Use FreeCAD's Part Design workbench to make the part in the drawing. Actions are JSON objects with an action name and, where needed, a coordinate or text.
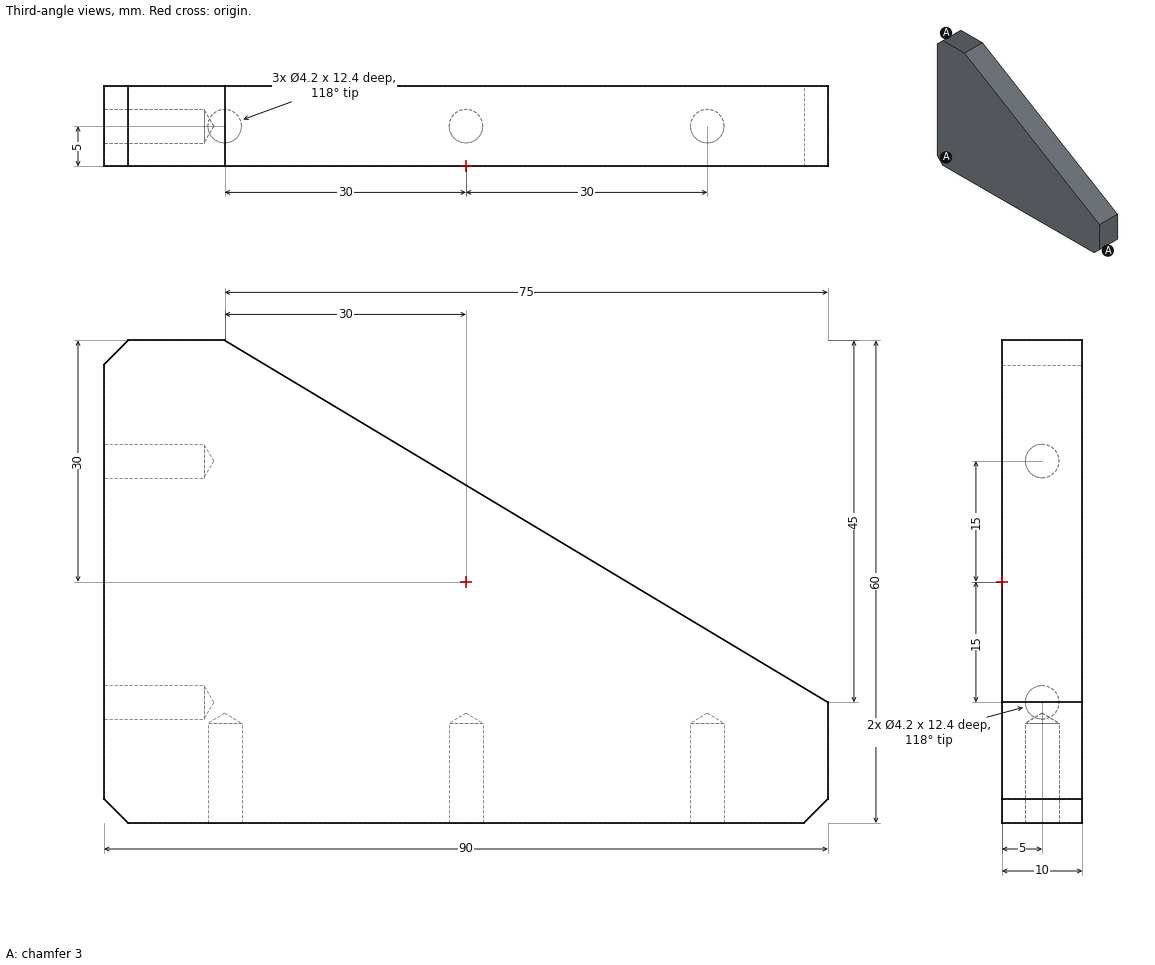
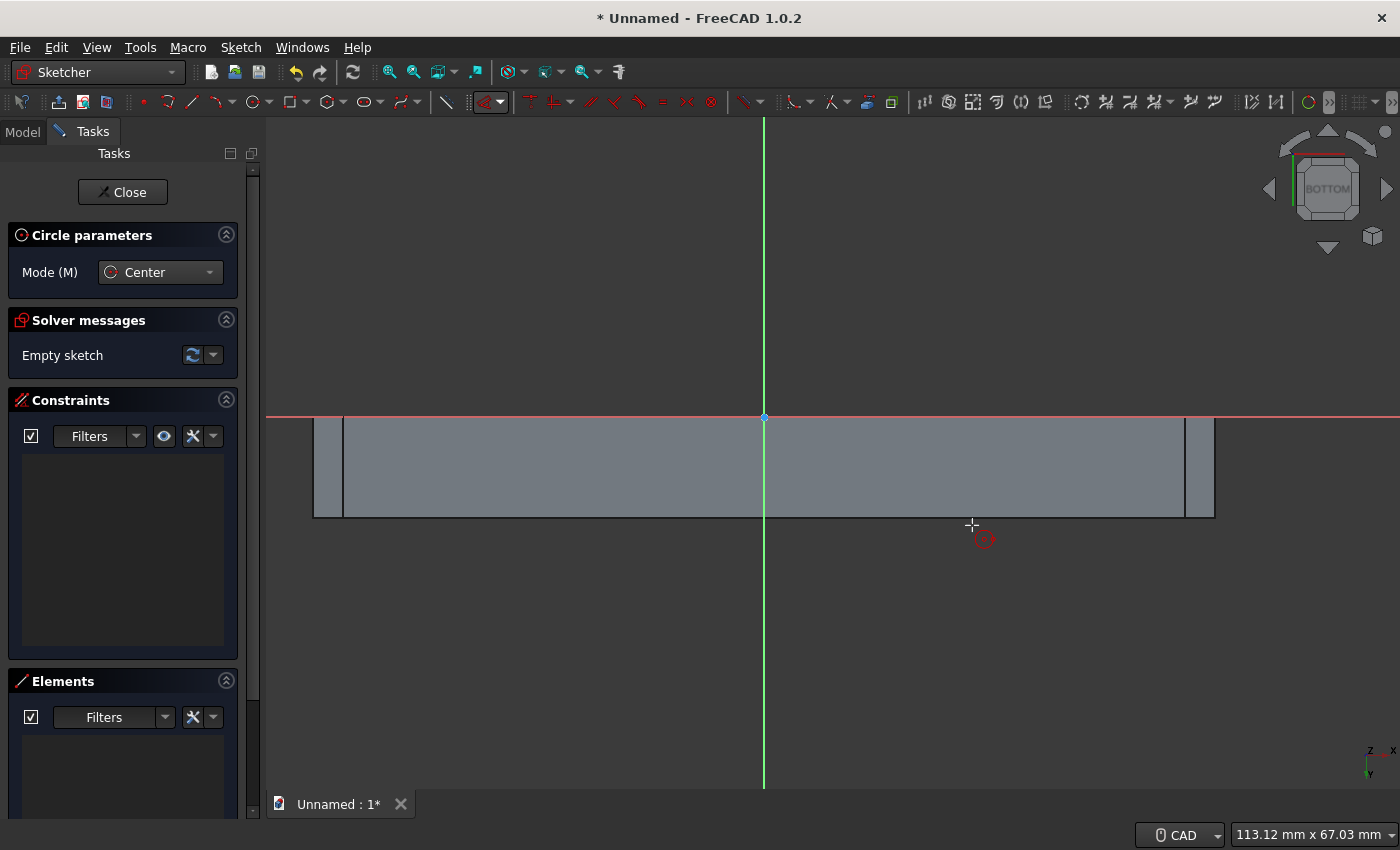
{"action": "left_click", "coordinate": [464, 467]}
{"action": "mouse_move", "coordinate": [478, 453]}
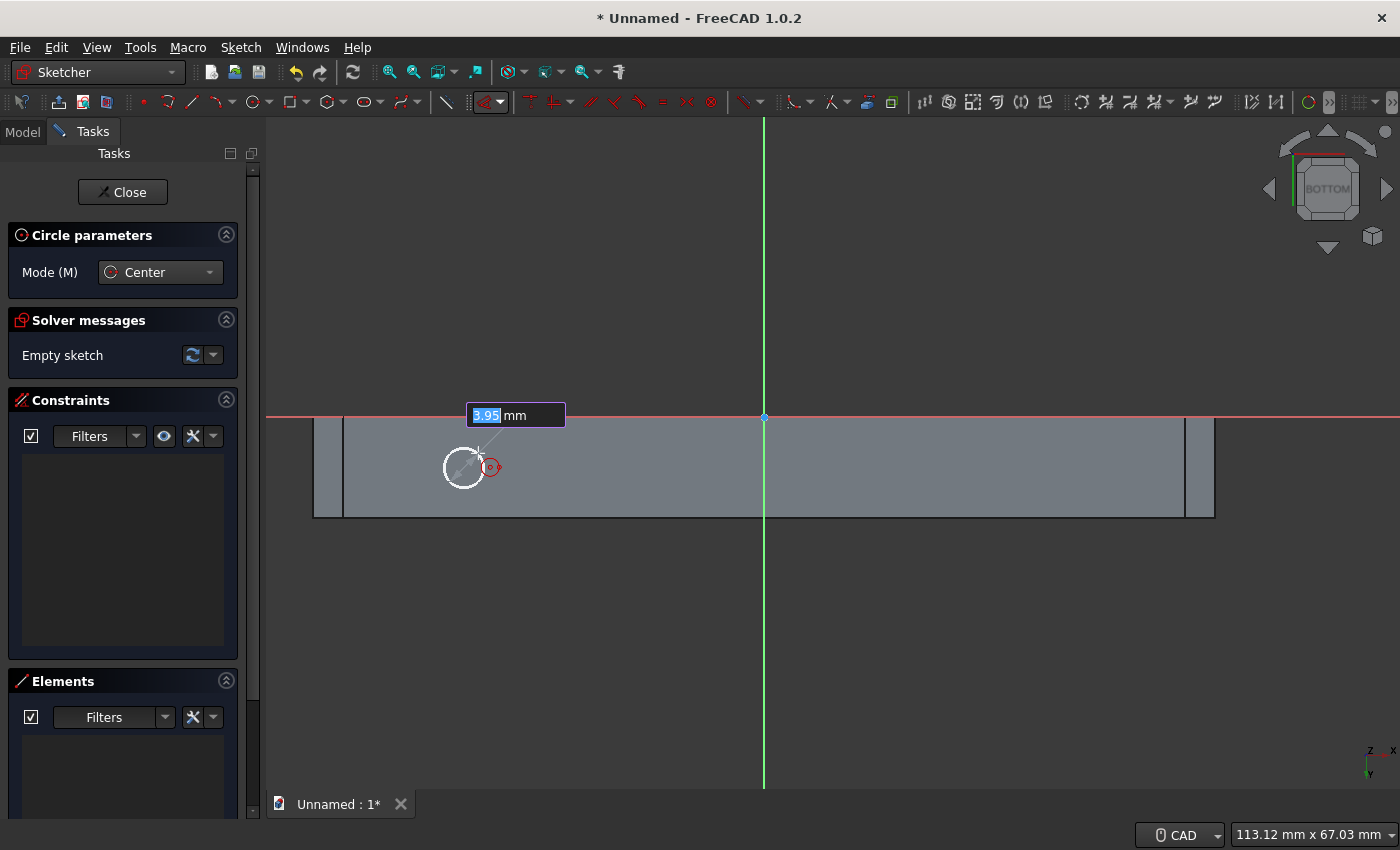
{"action": "type", "text": "4.2"}
{"action": "key", "text": "Return"}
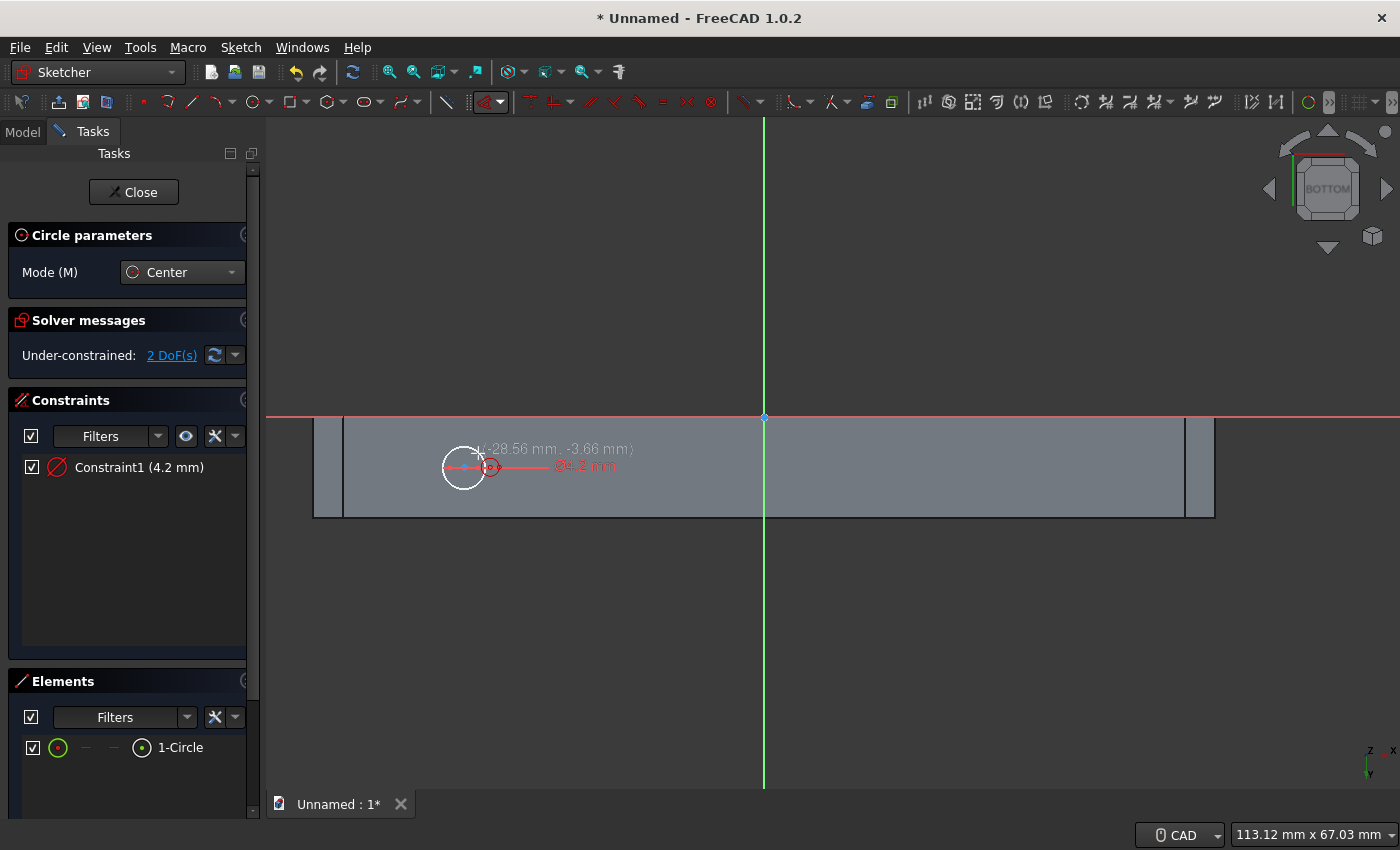
{"action": "left_click", "coordinate": [764, 467]}
{"action": "mouse_move", "coordinate": [779, 453]}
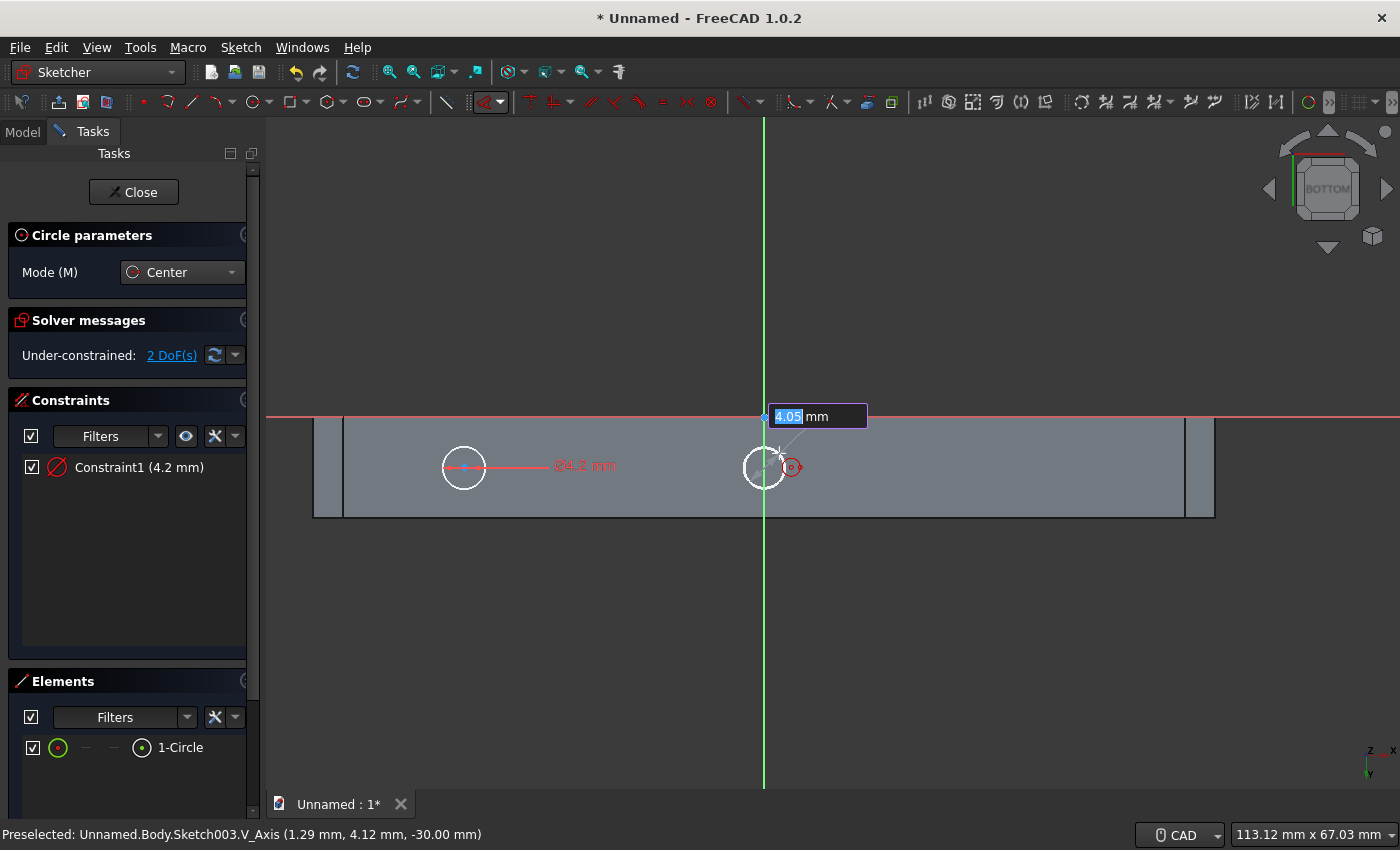
{"action": "type", "text": "4.2"}
{"action": "key", "text": "Return"}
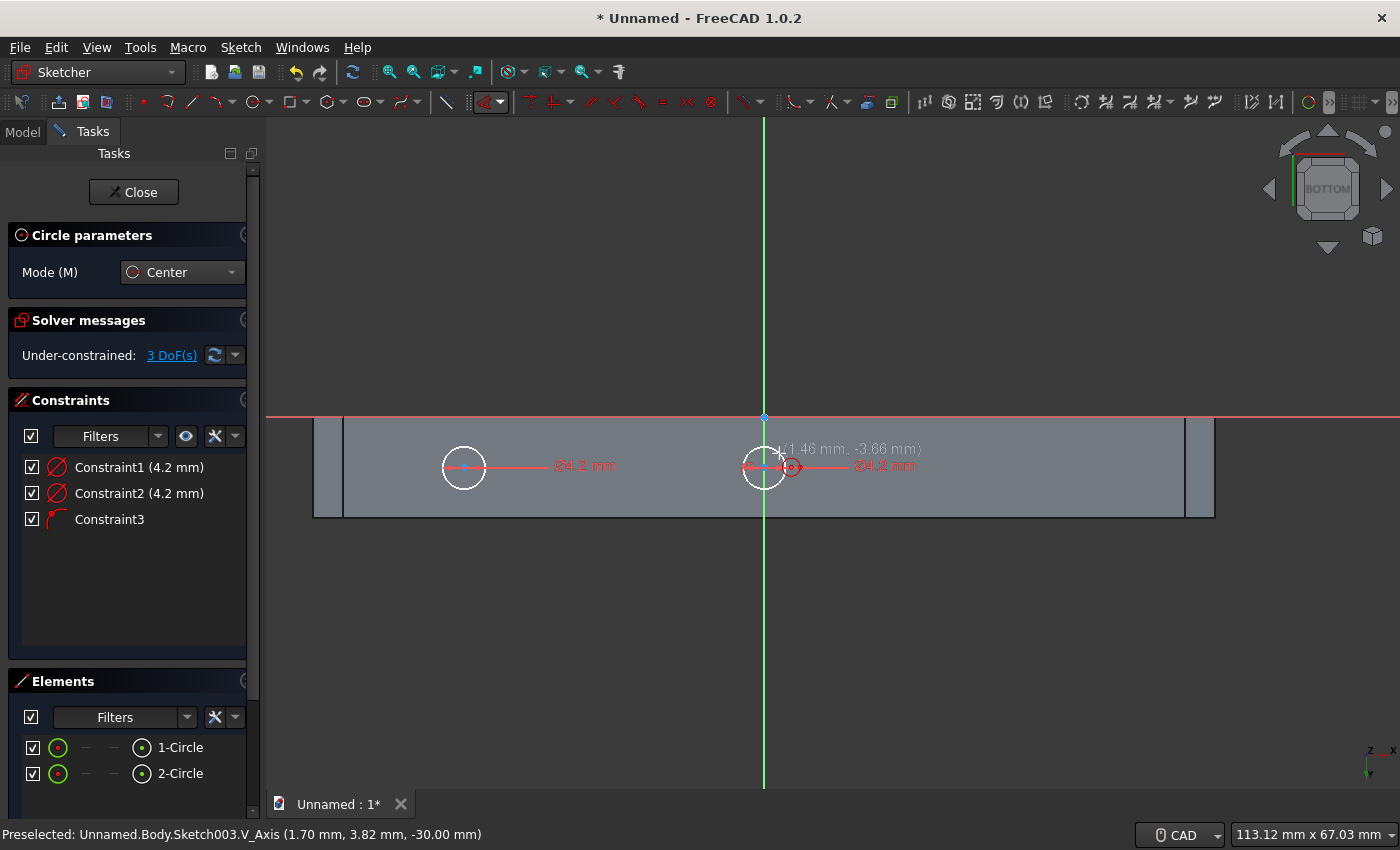
{"action": "left_click", "coordinate": [1065, 467]}
{"action": "mouse_move", "coordinate": [1080, 453]}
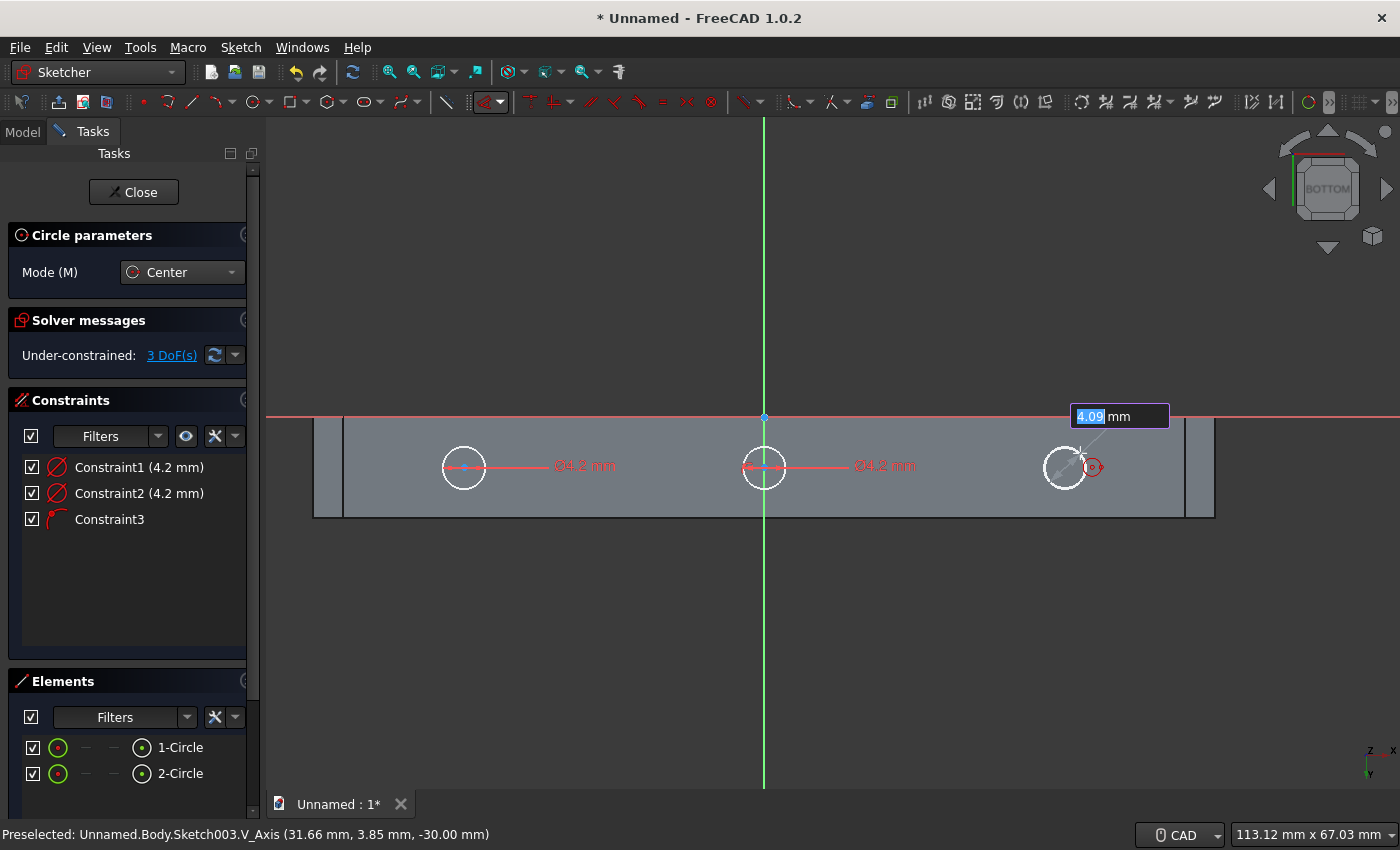
{"action": "type", "text": "4.2"}
{"action": "key", "text": "Return"}
{"action": "key", "text": "Escape"}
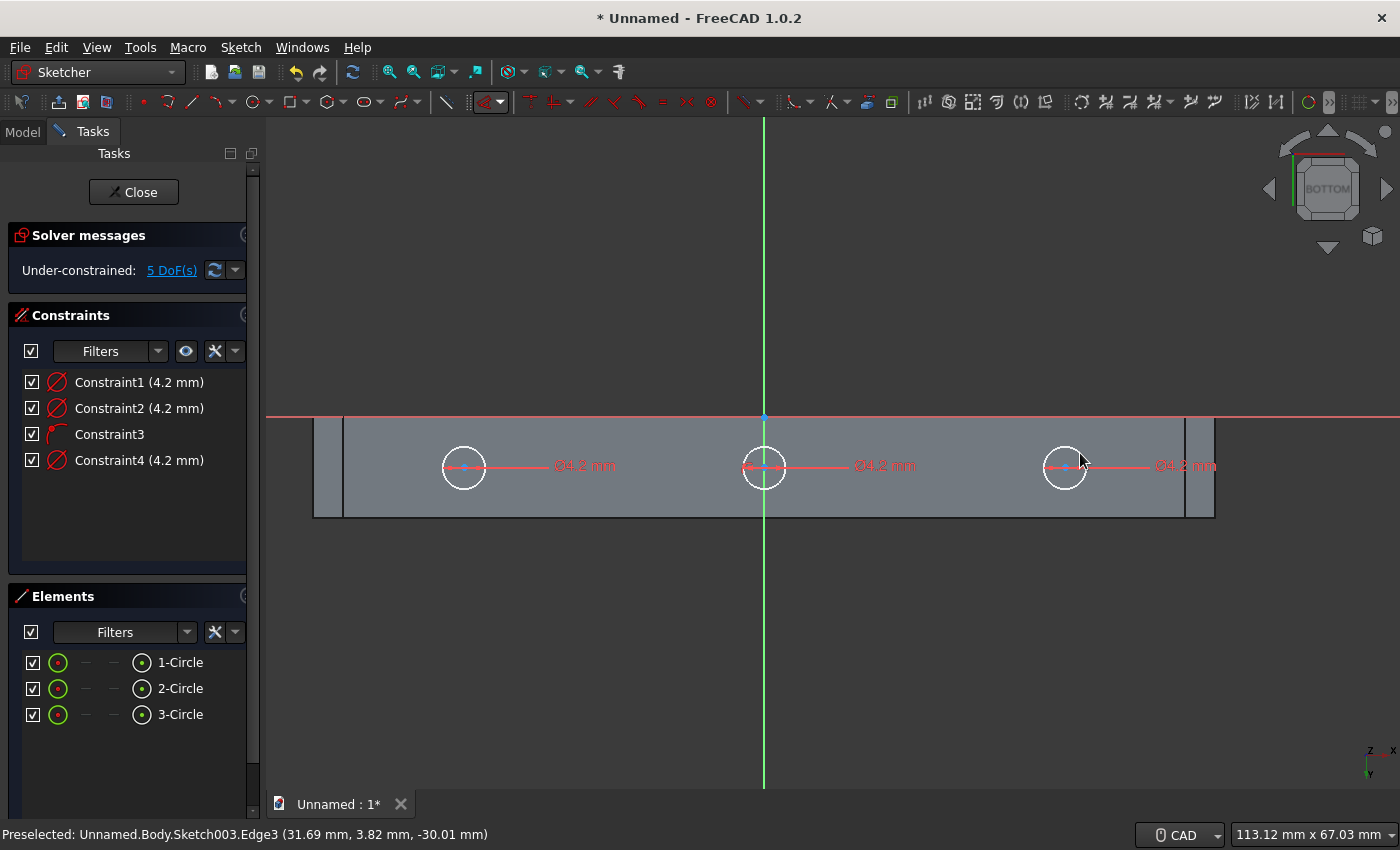
{"action": "left_click", "coordinate": [464, 468]}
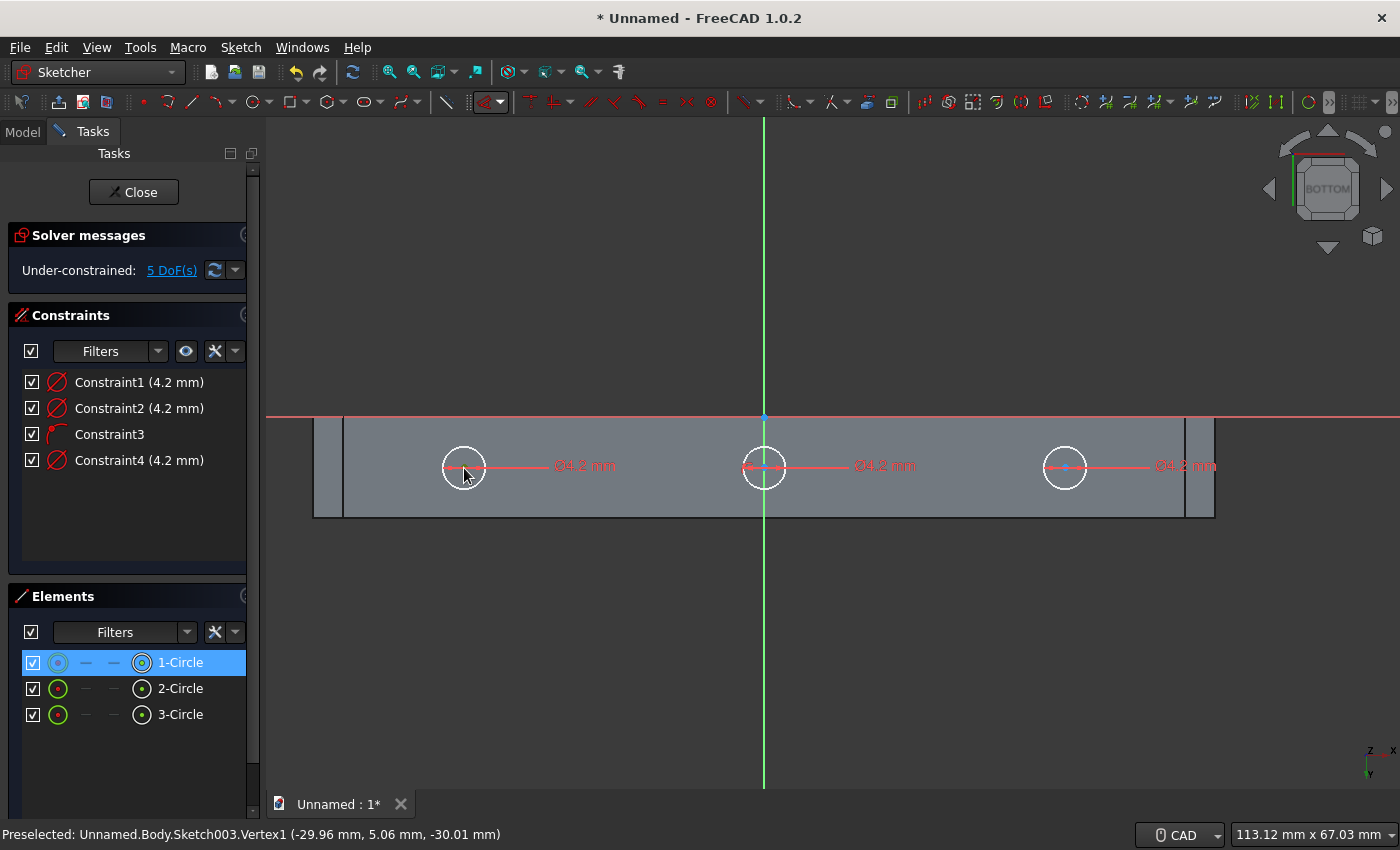
{"action": "left_click", "coordinate": [764, 468]}